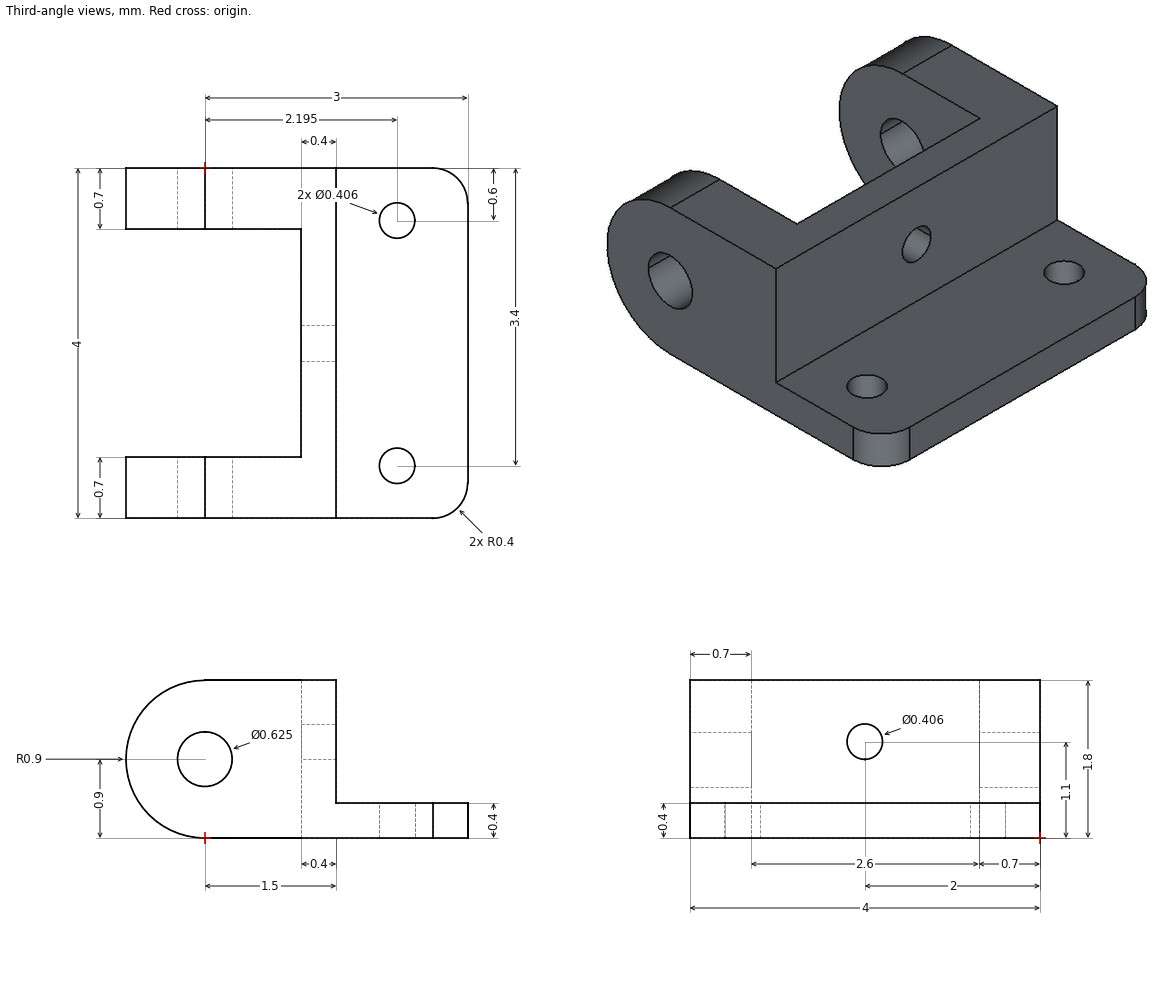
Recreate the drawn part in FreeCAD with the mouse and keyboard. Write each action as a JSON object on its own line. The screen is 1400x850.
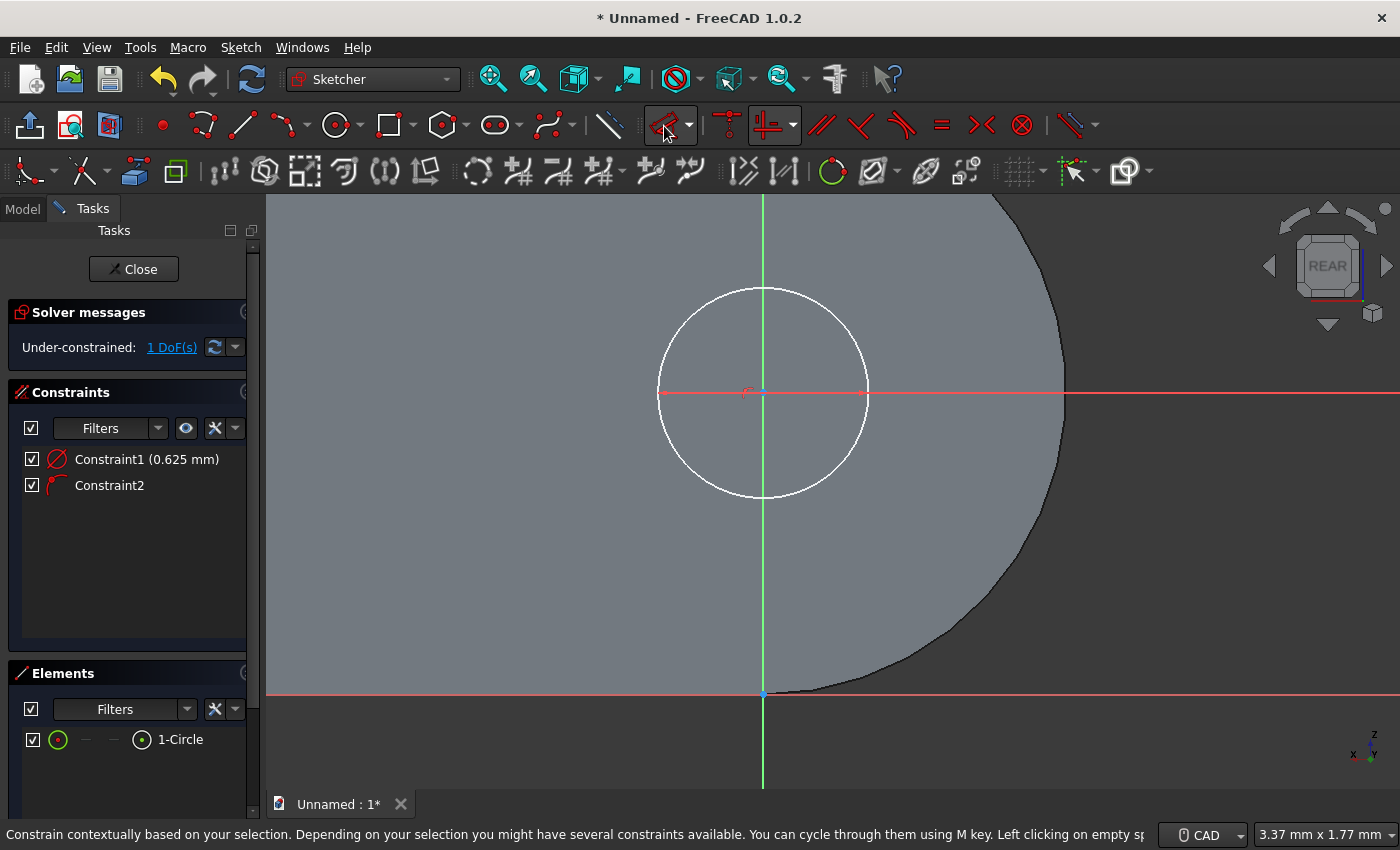
{"action": "scroll", "coordinate": [763, 393], "scroll_direction": "up", "scroll_amount": 4}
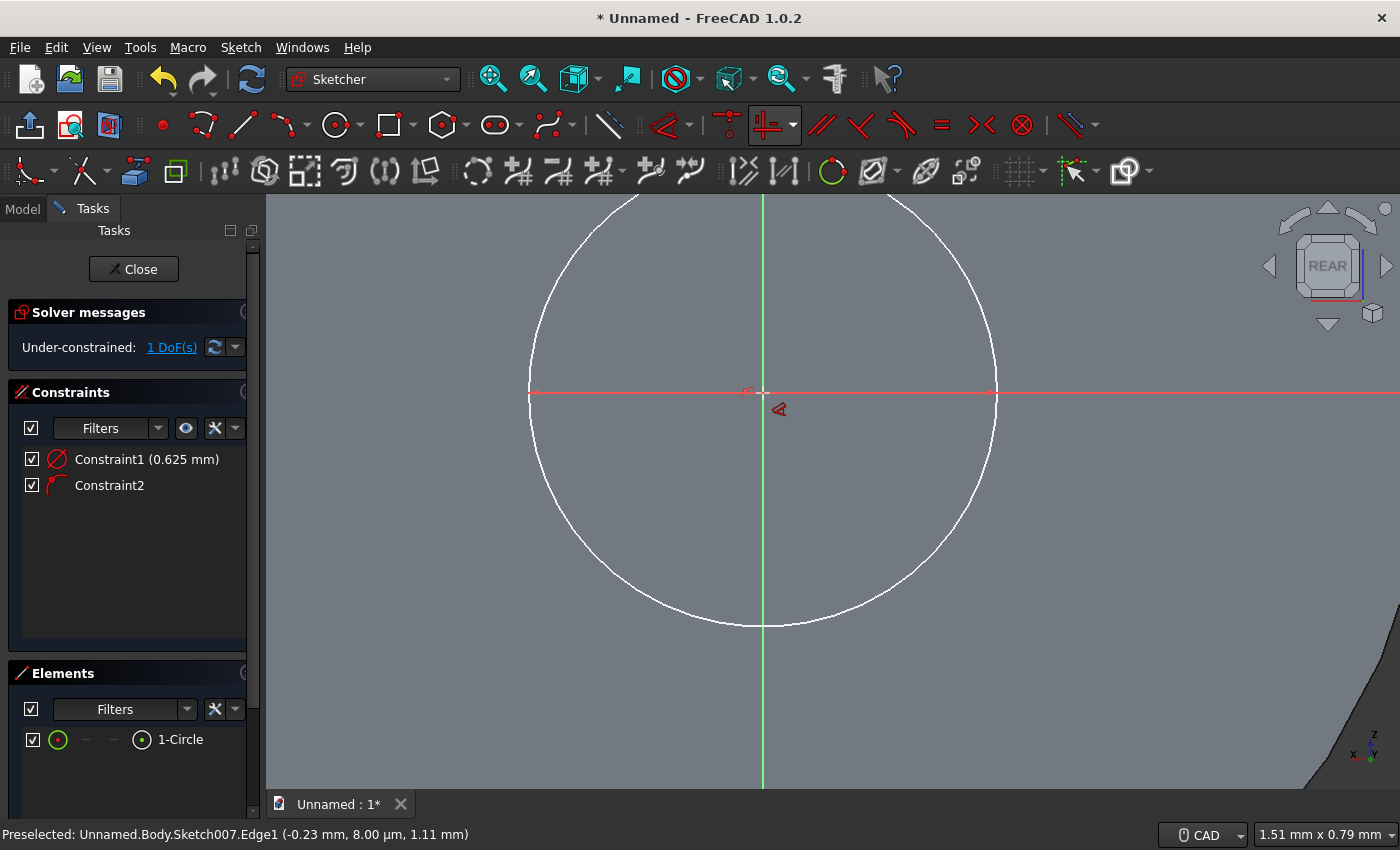
{"action": "left_click", "coordinate": [763, 393]}
{"action": "left_click", "coordinate": [797, 577]}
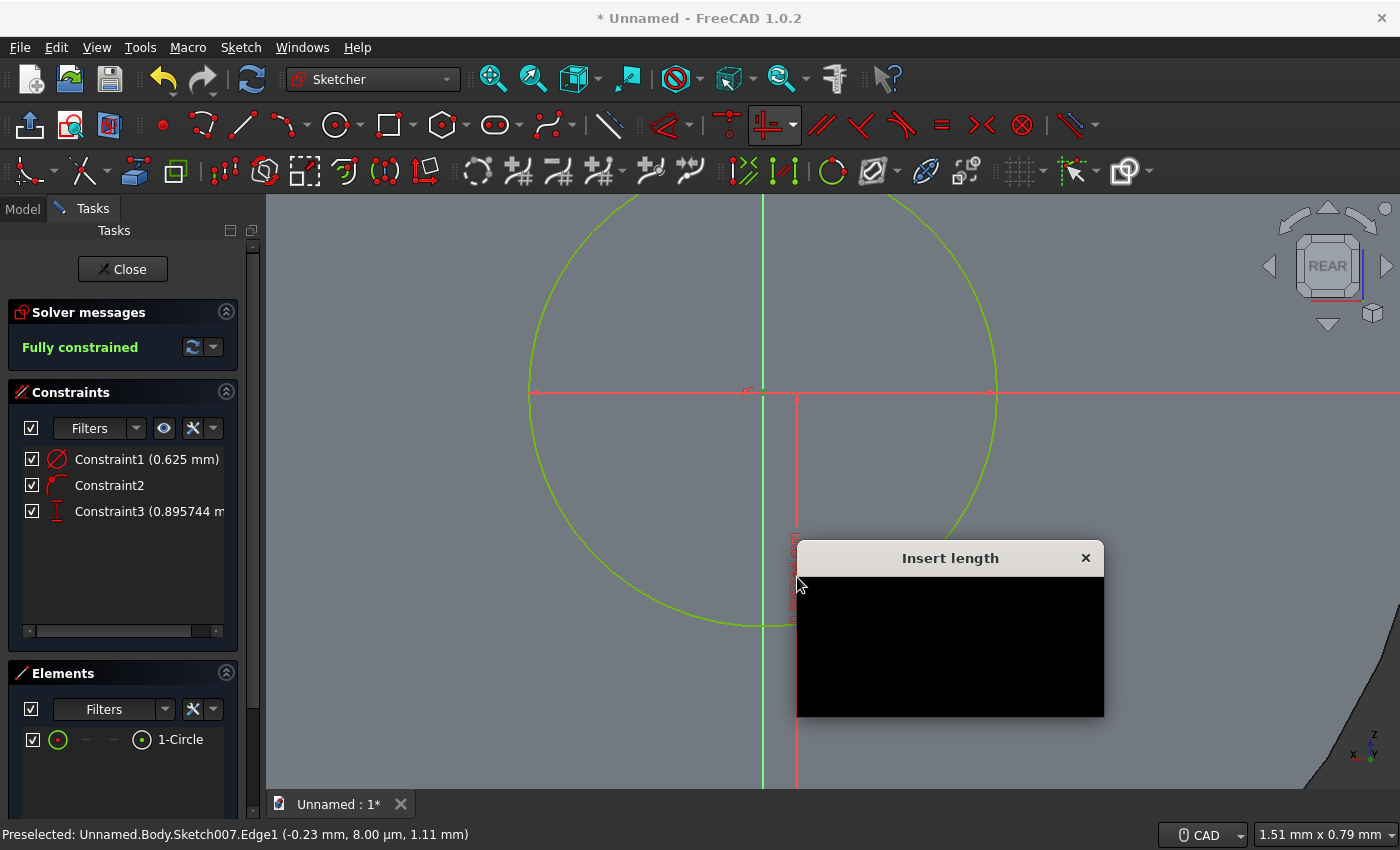
{"action": "type", "text": "0.9"}
{"action": "key", "text": "Return"}
{"action": "key", "text": "Escape"}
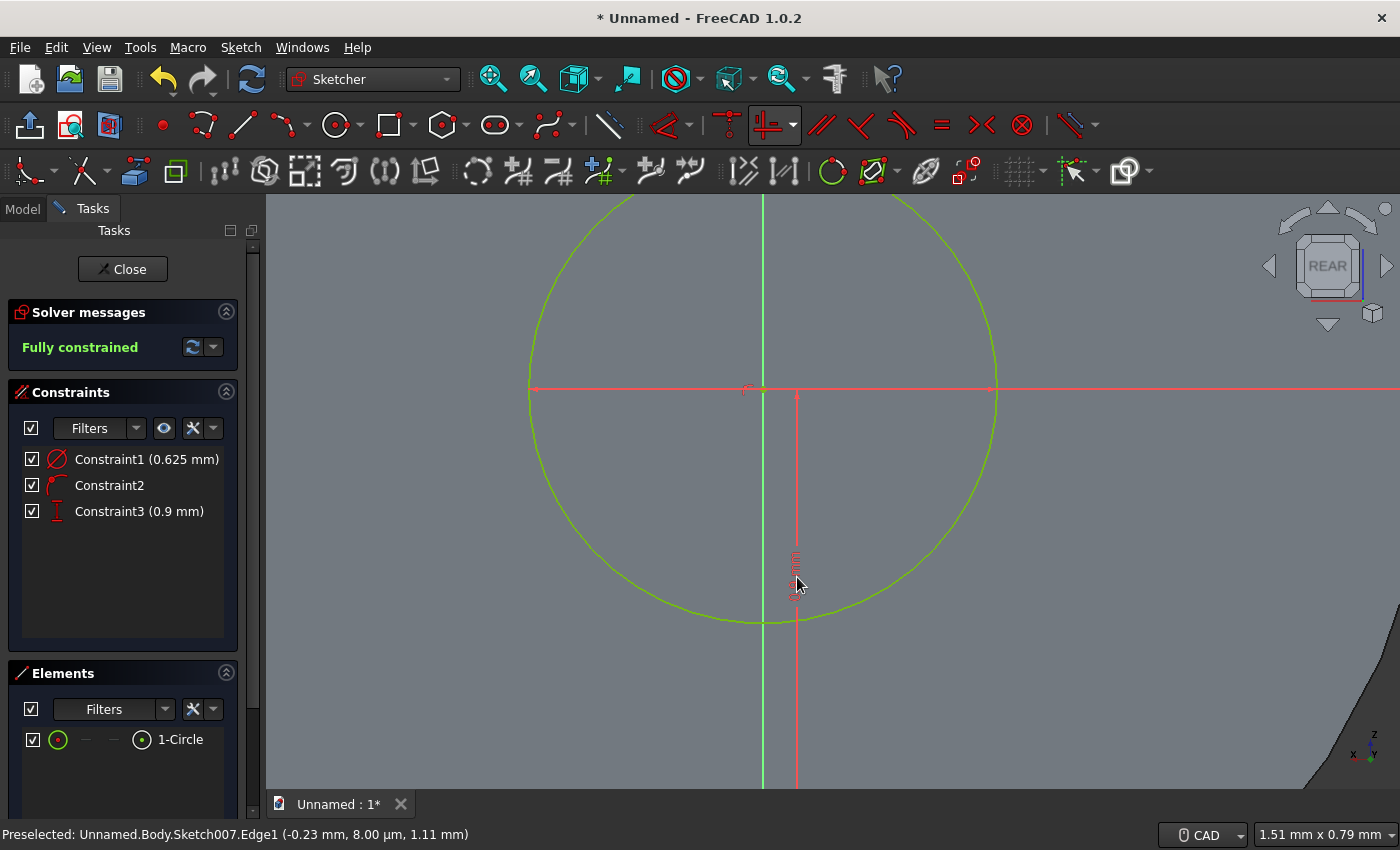
{"action": "left_click", "coordinate": [123, 269]}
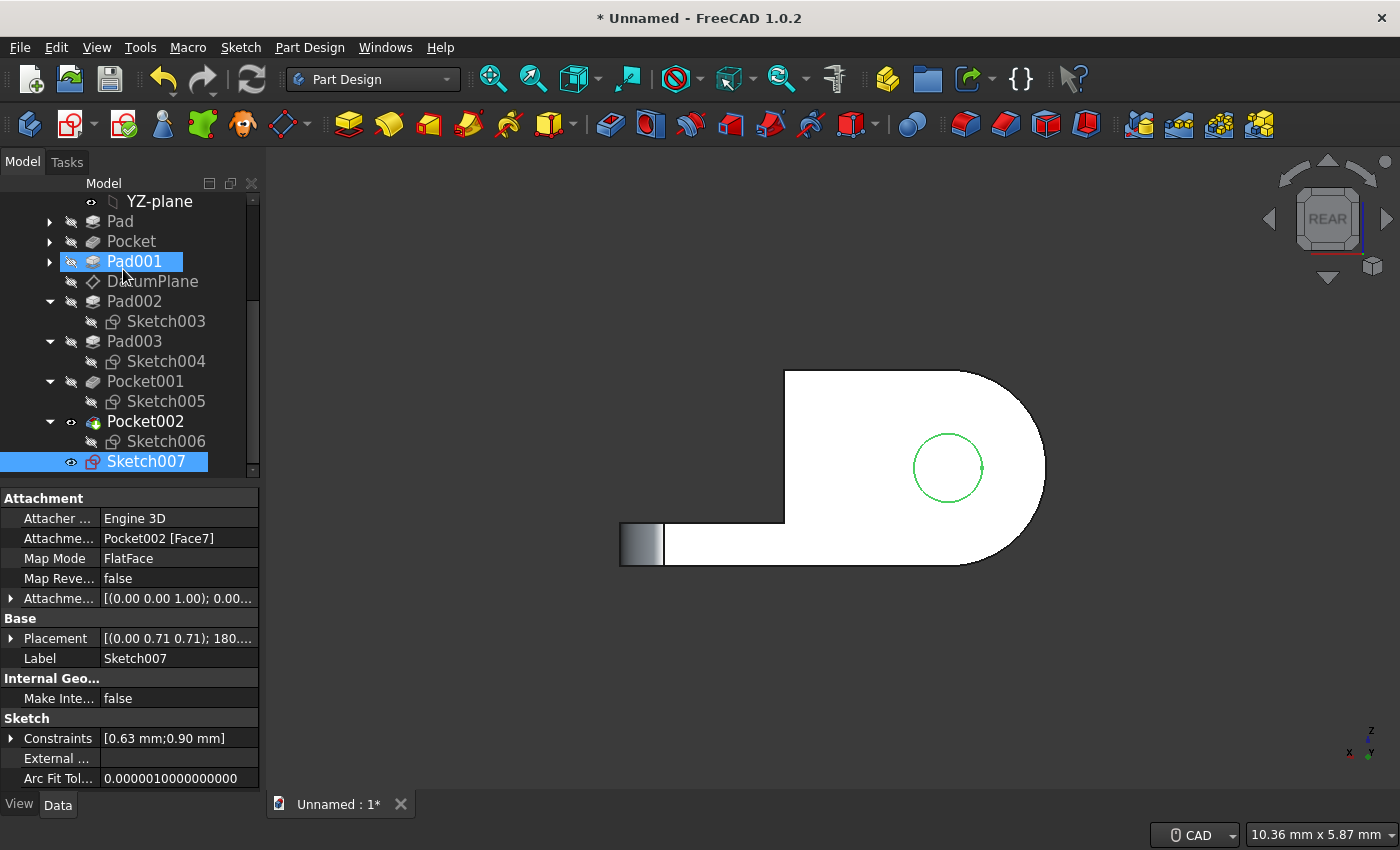
{"action": "left_click", "coordinate": [612, 124]}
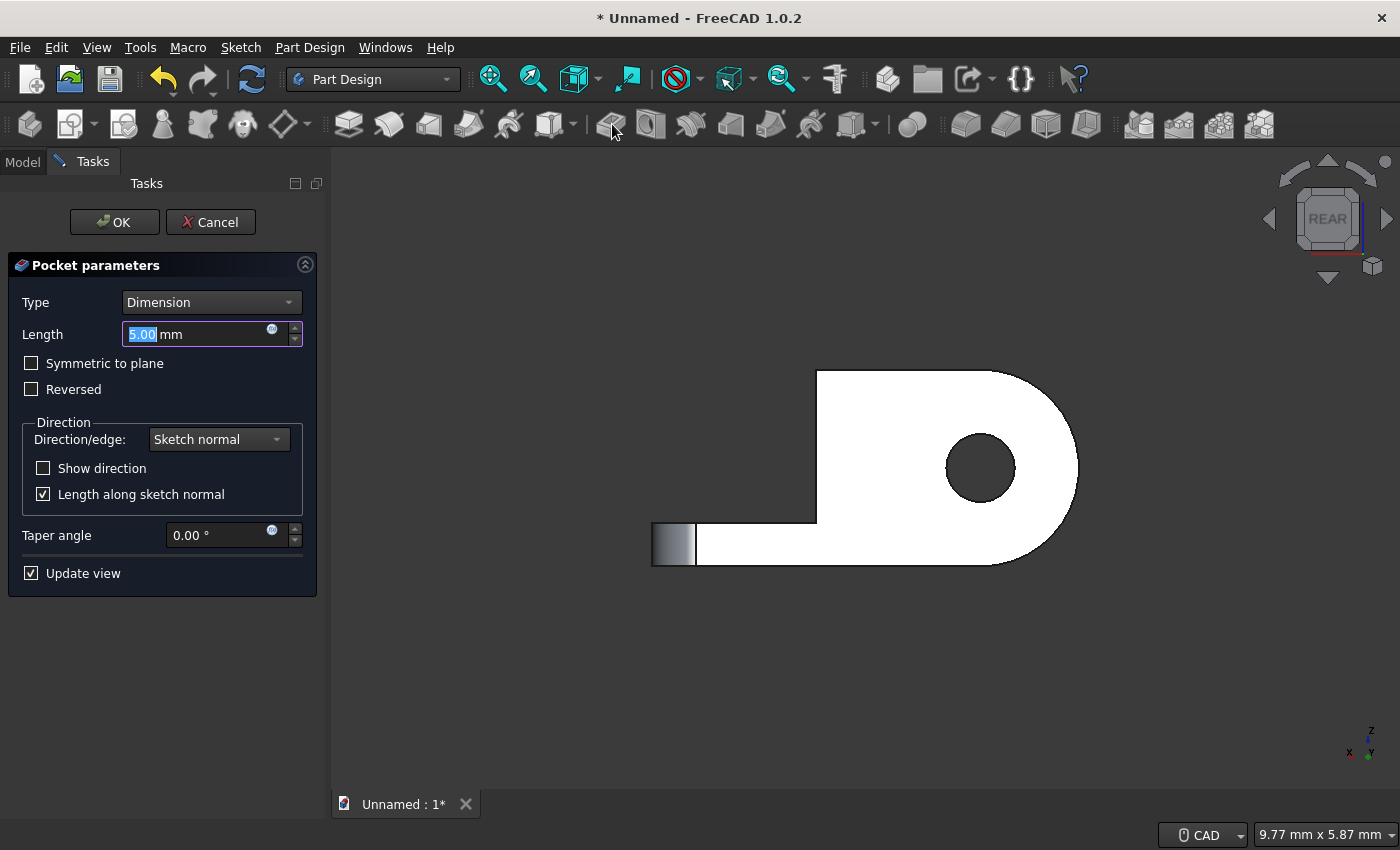
{"action": "type", "text": "0.7"}
{"action": "key", "text": "Tab"}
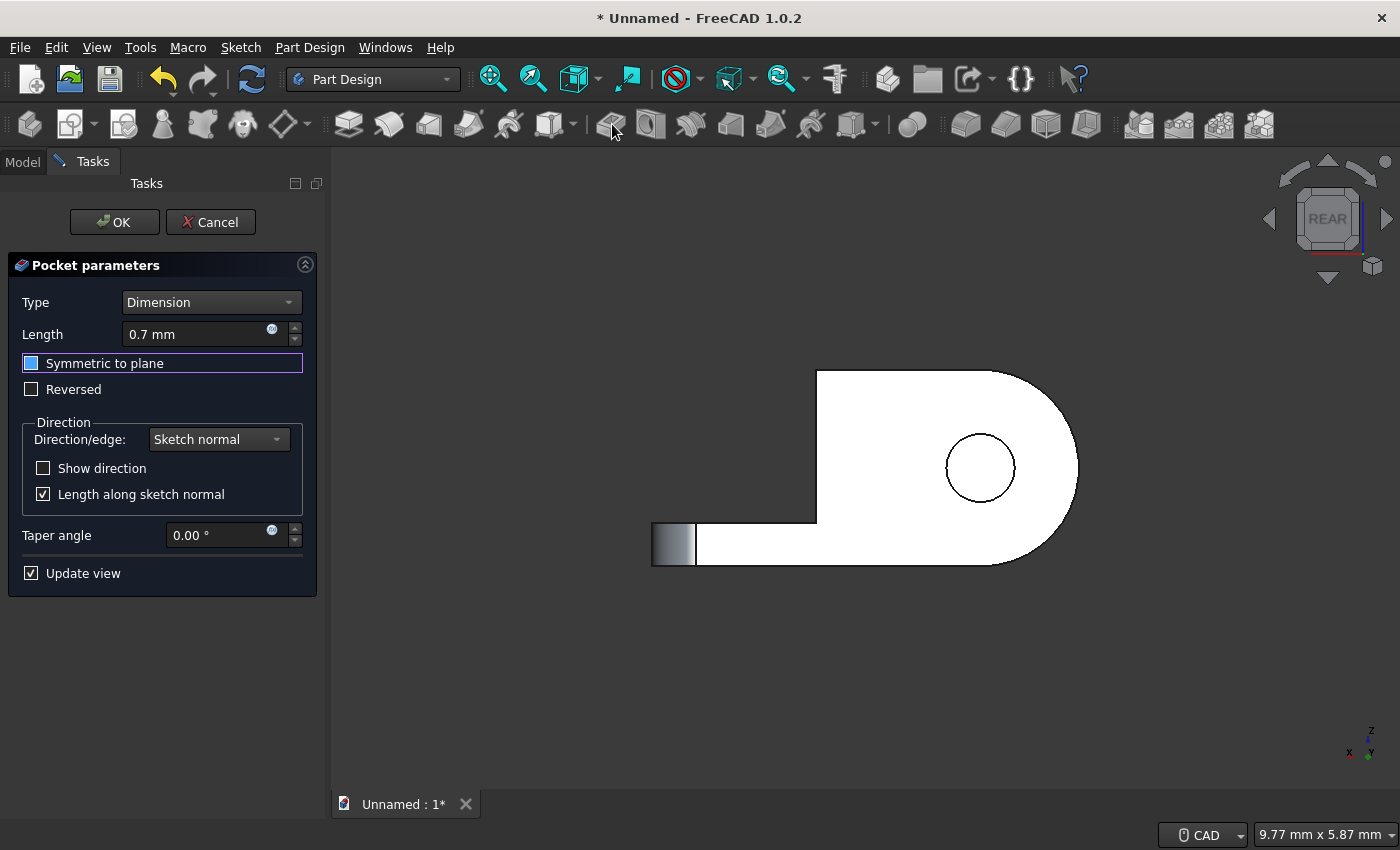
{"action": "left_click", "coordinate": [115, 222]}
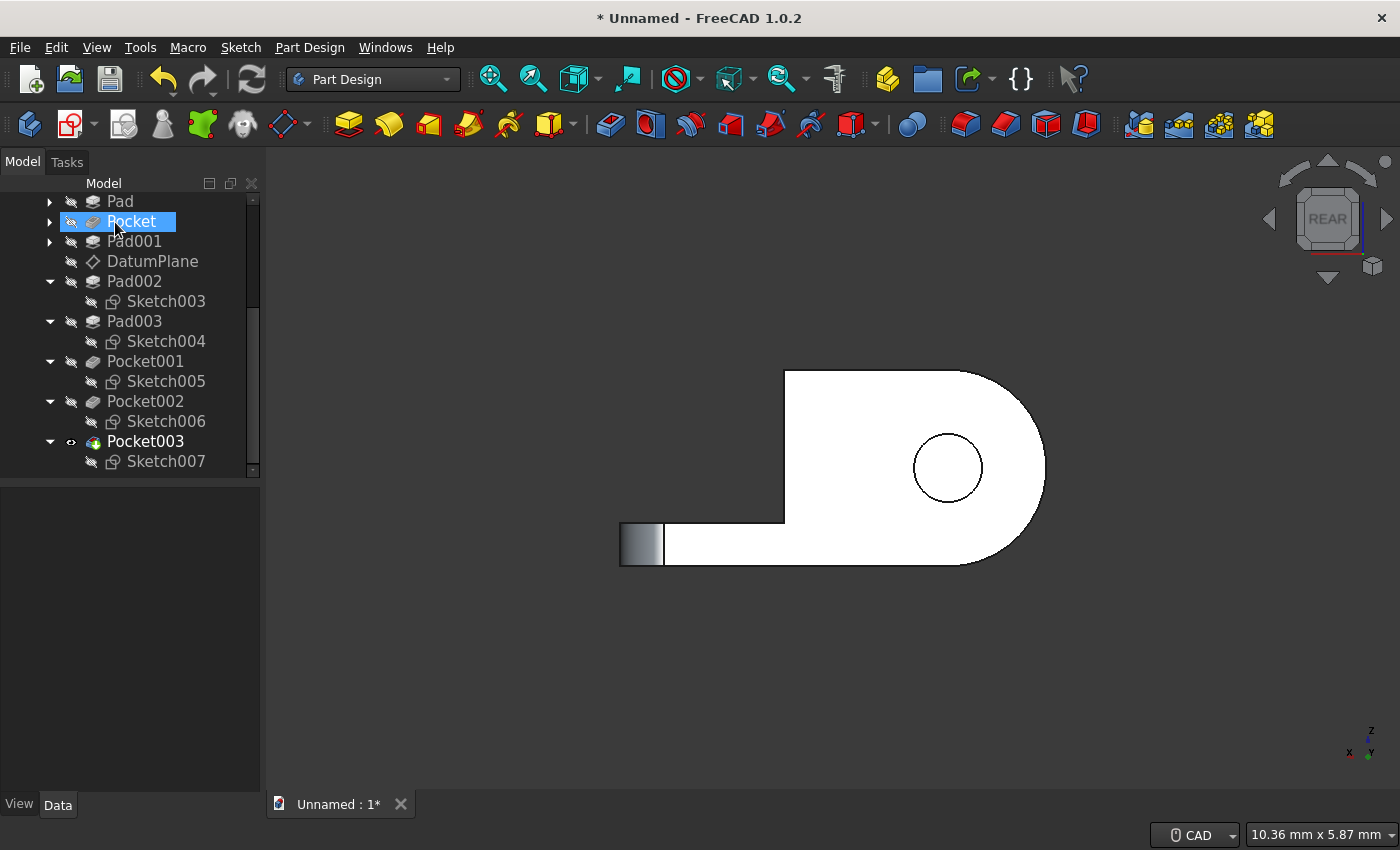
{"action": "key", "text": "v f"}